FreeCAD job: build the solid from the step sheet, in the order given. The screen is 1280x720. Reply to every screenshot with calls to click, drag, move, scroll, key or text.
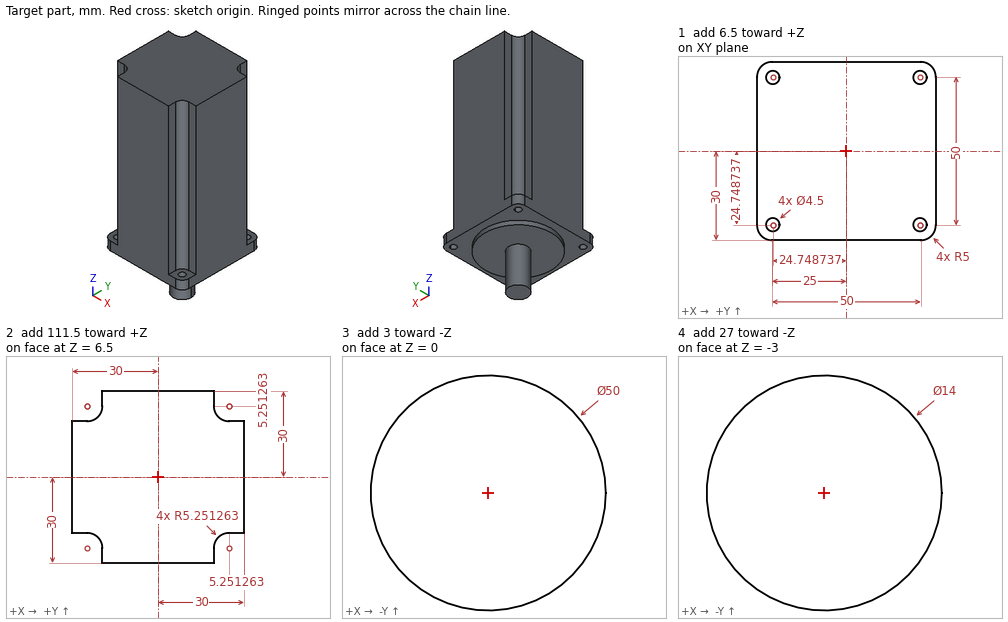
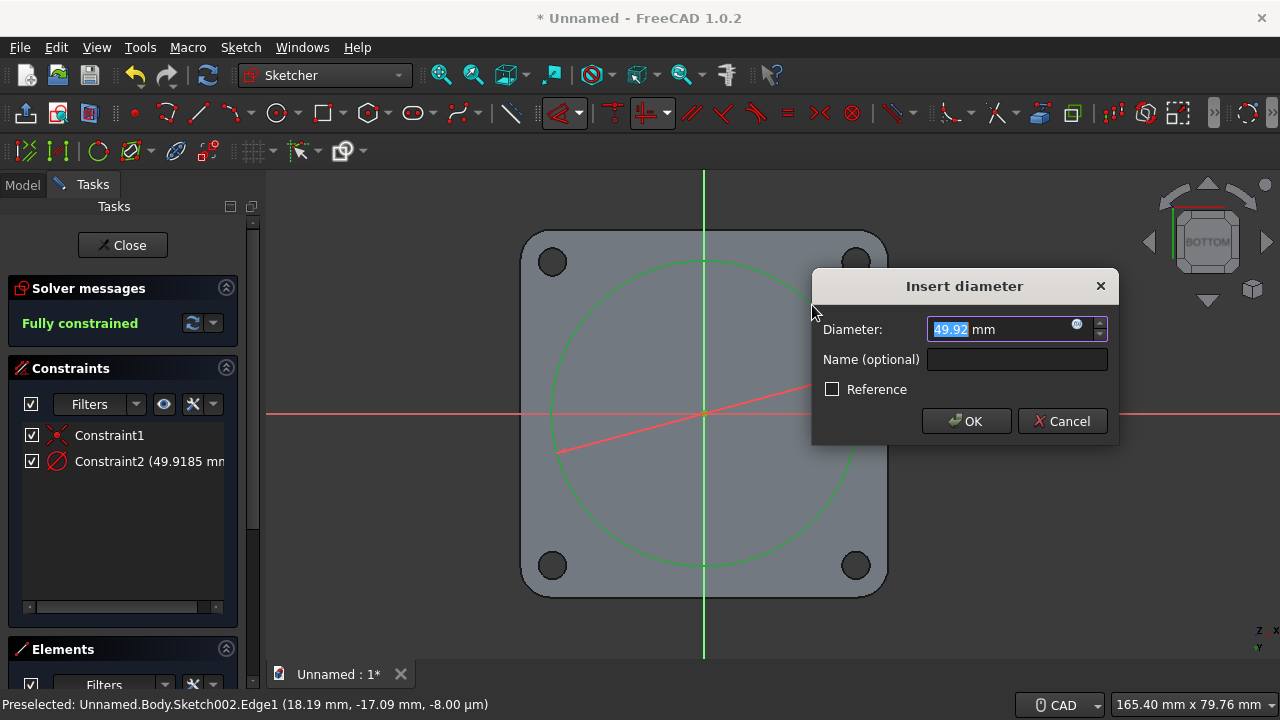
text(50)
key(Return)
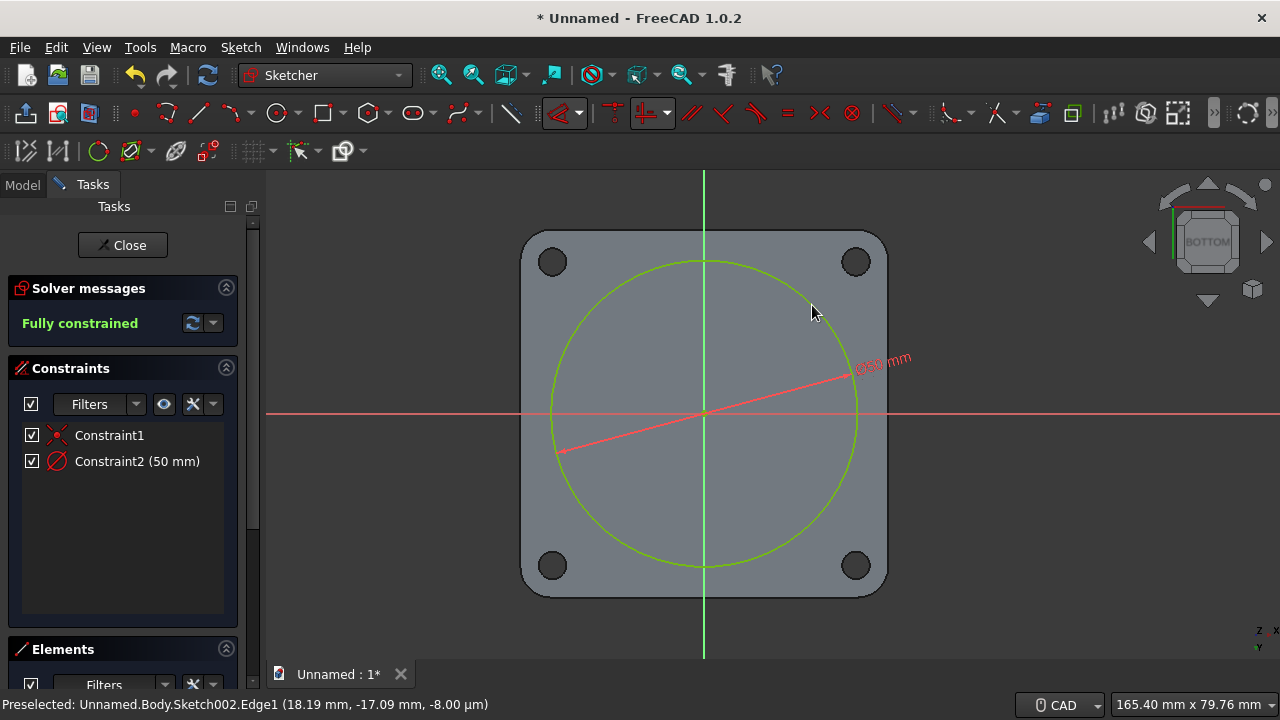
click(123, 245)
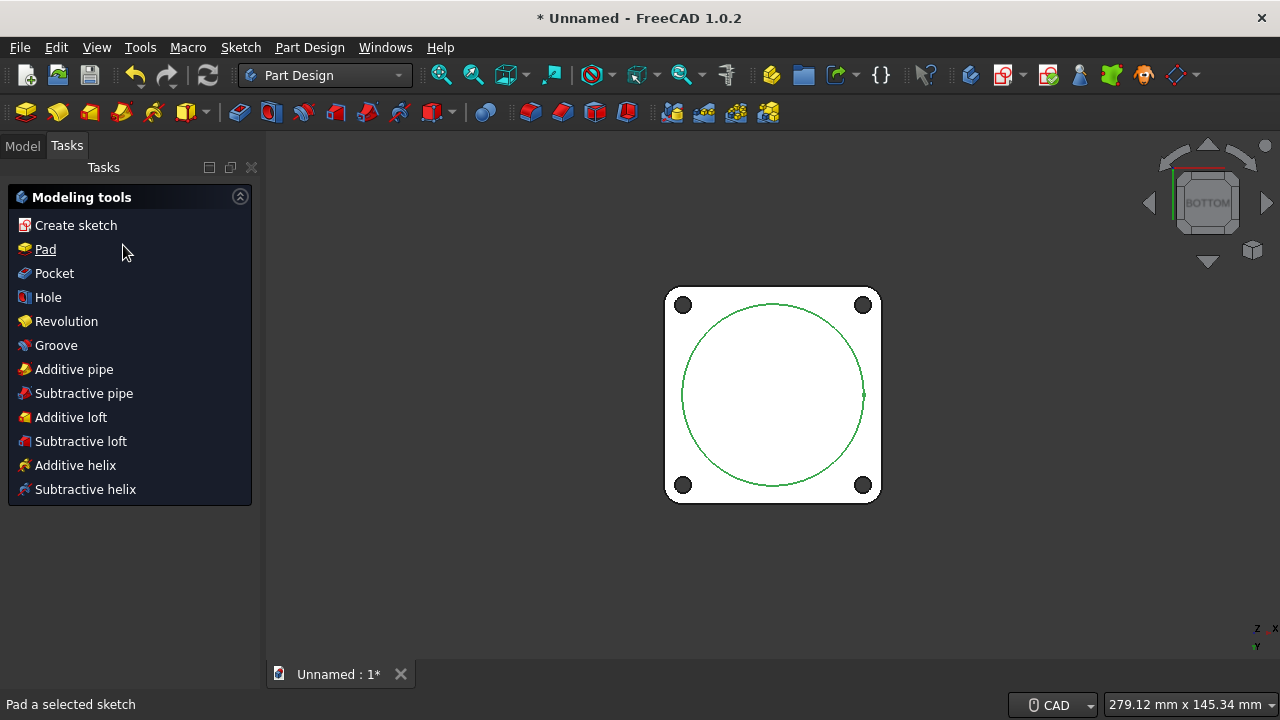
click(26, 112)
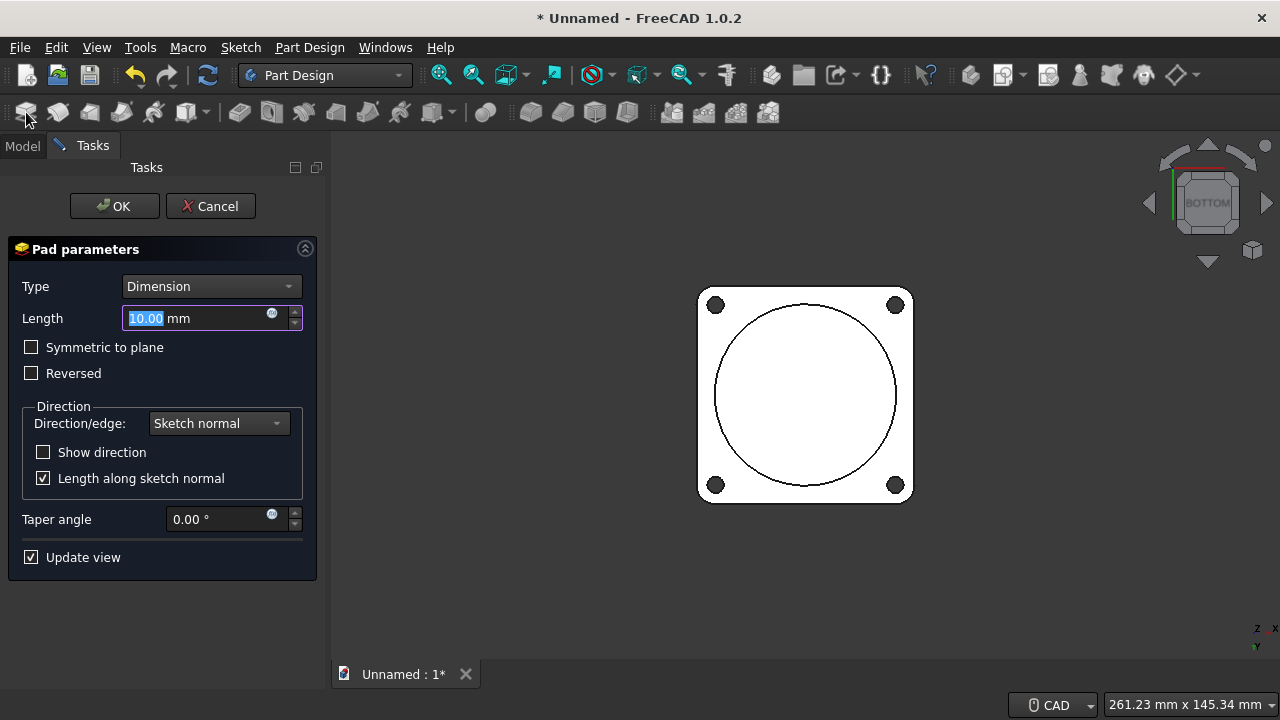
text(3)
key(Tab)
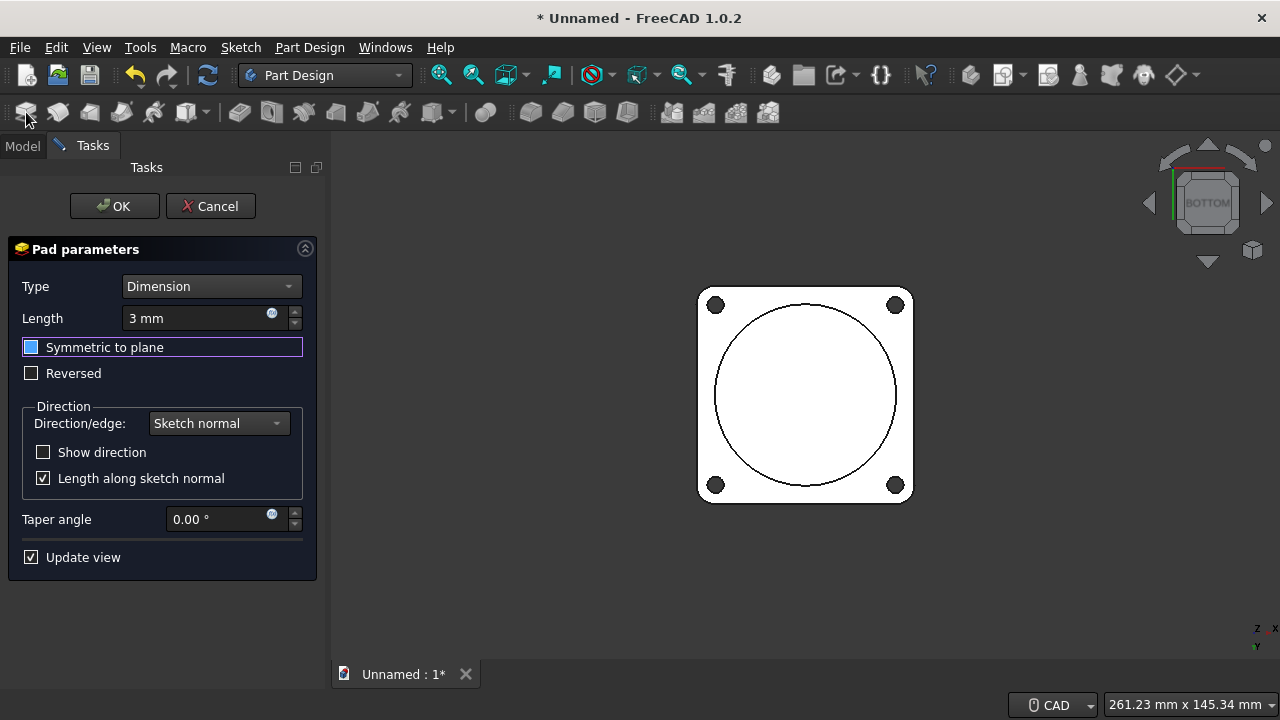
click(115, 206)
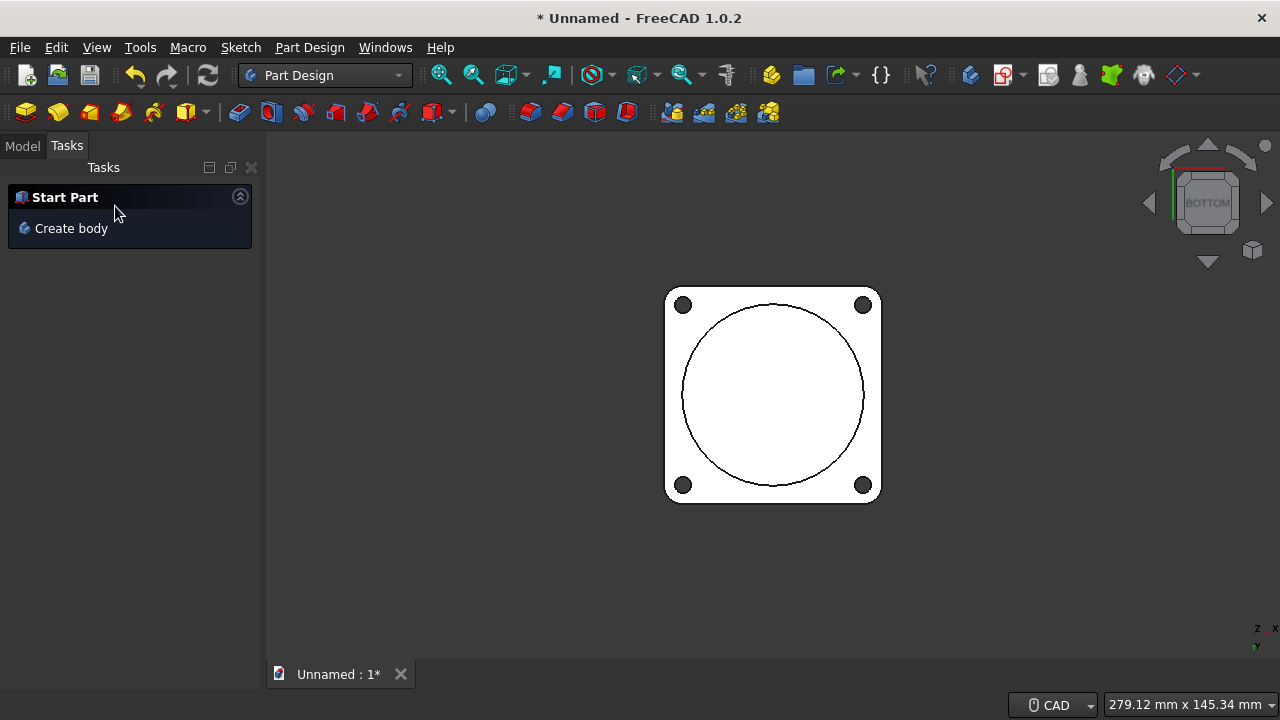
click(442, 76)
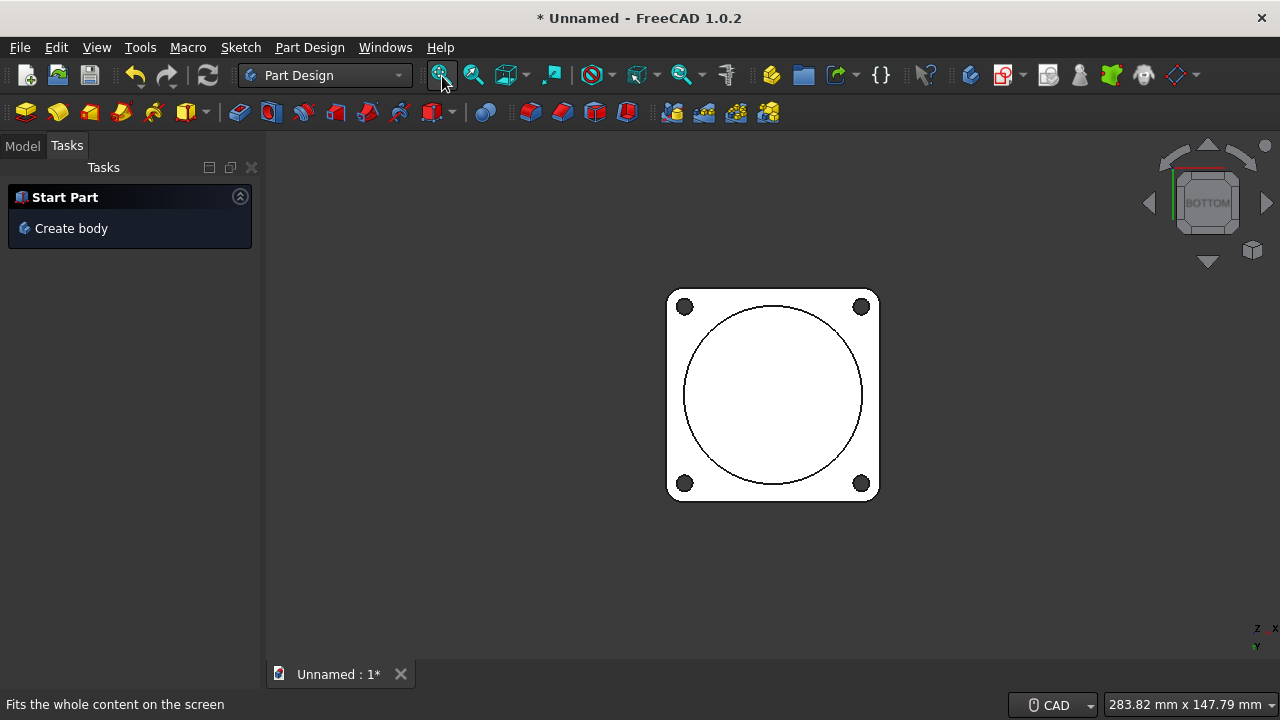
click(773, 394)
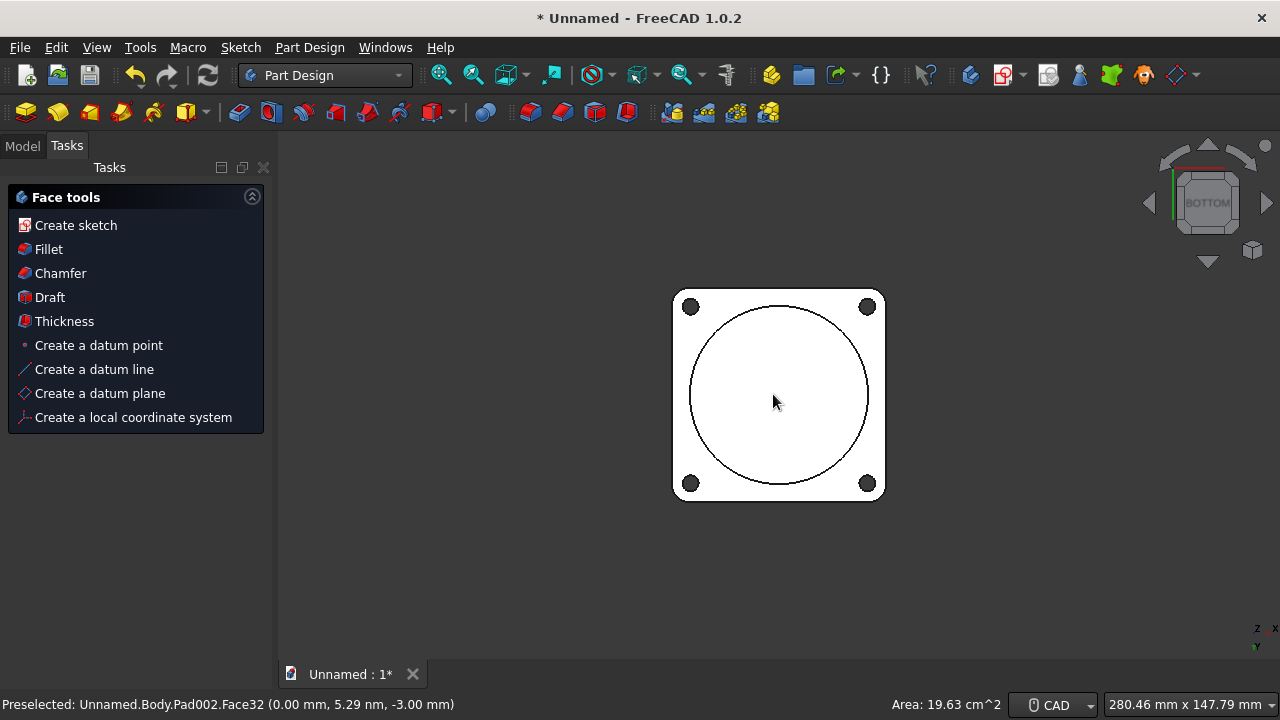
click(1004, 76)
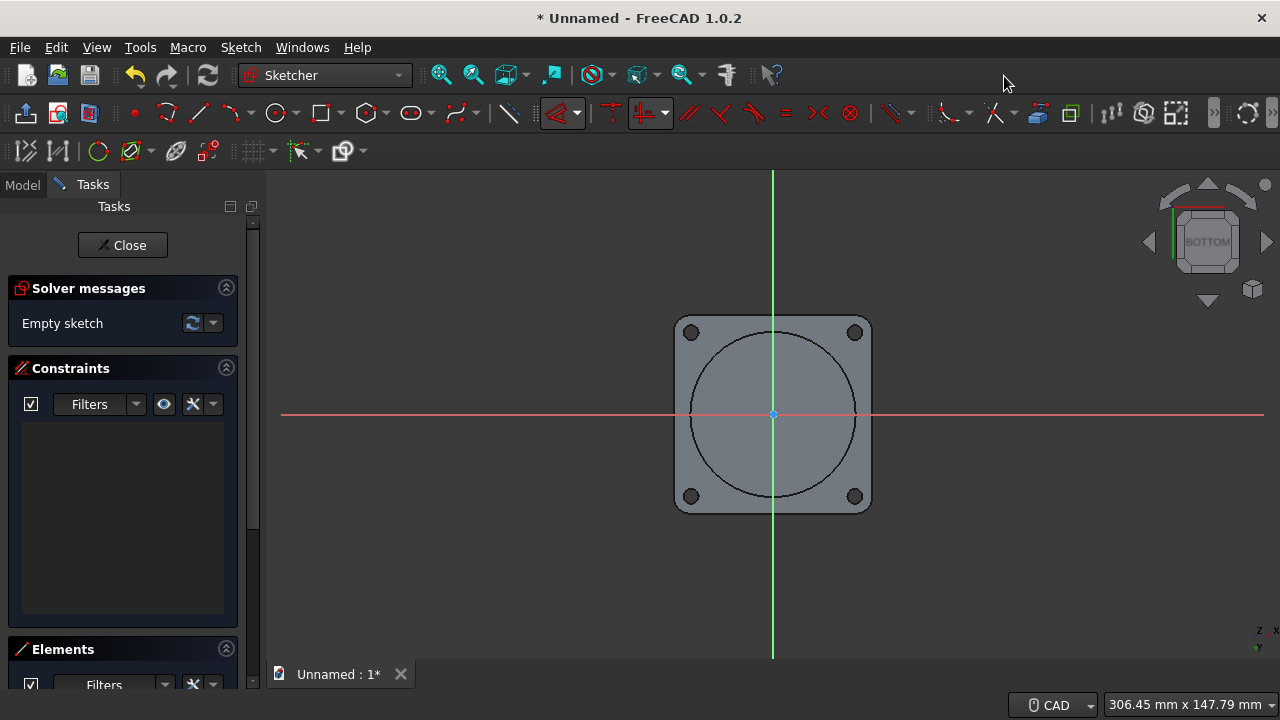
scroll(787, 414, up, 9)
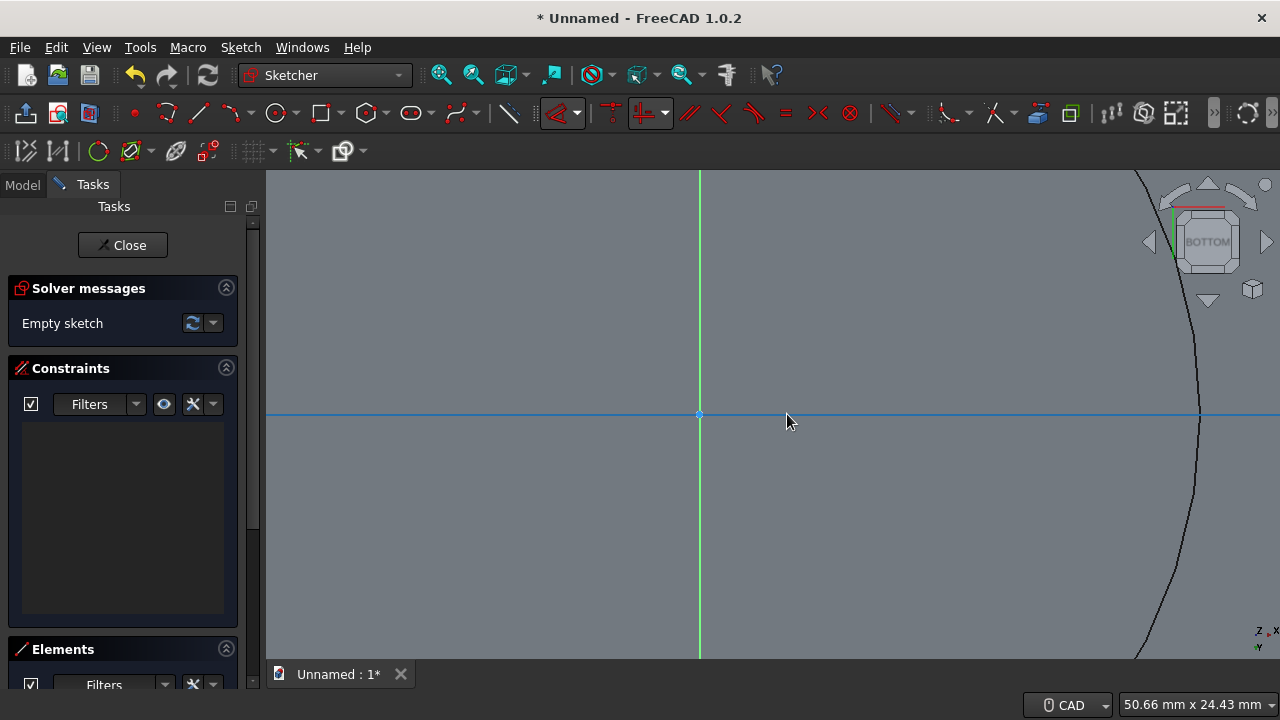
key(g)
key(c)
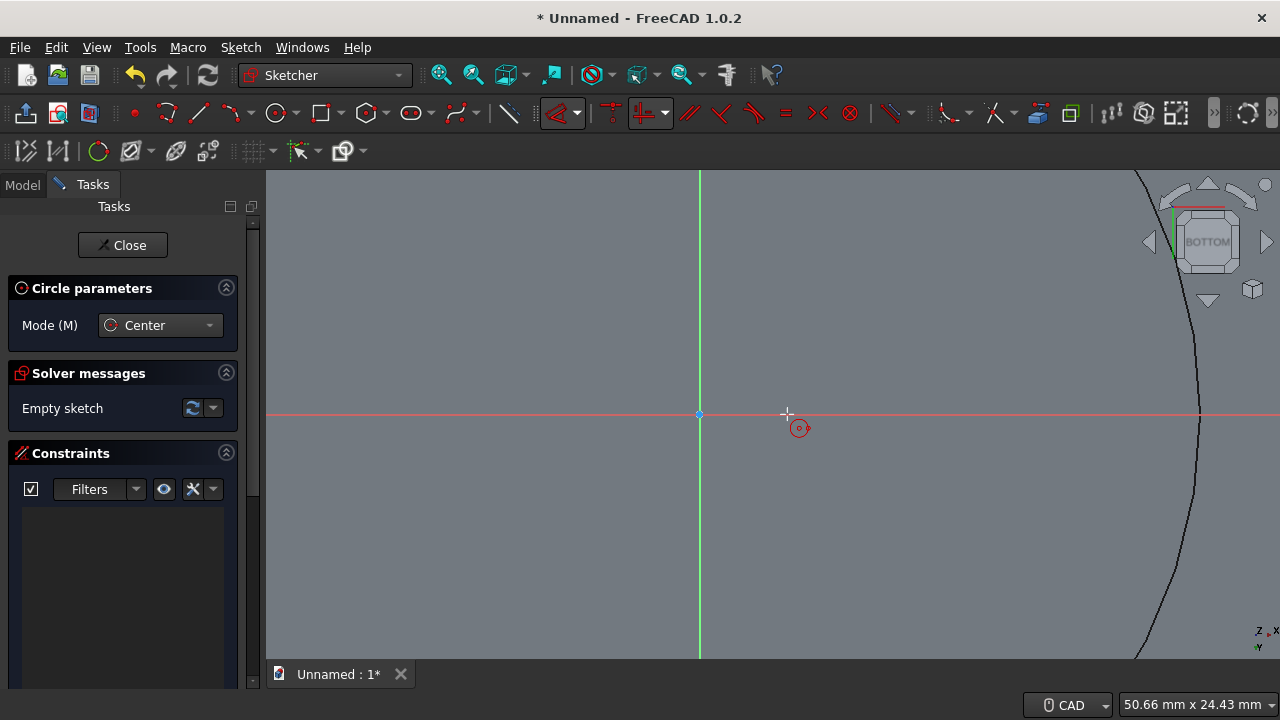
click(700, 414)
click(799, 315)
key(Escape)